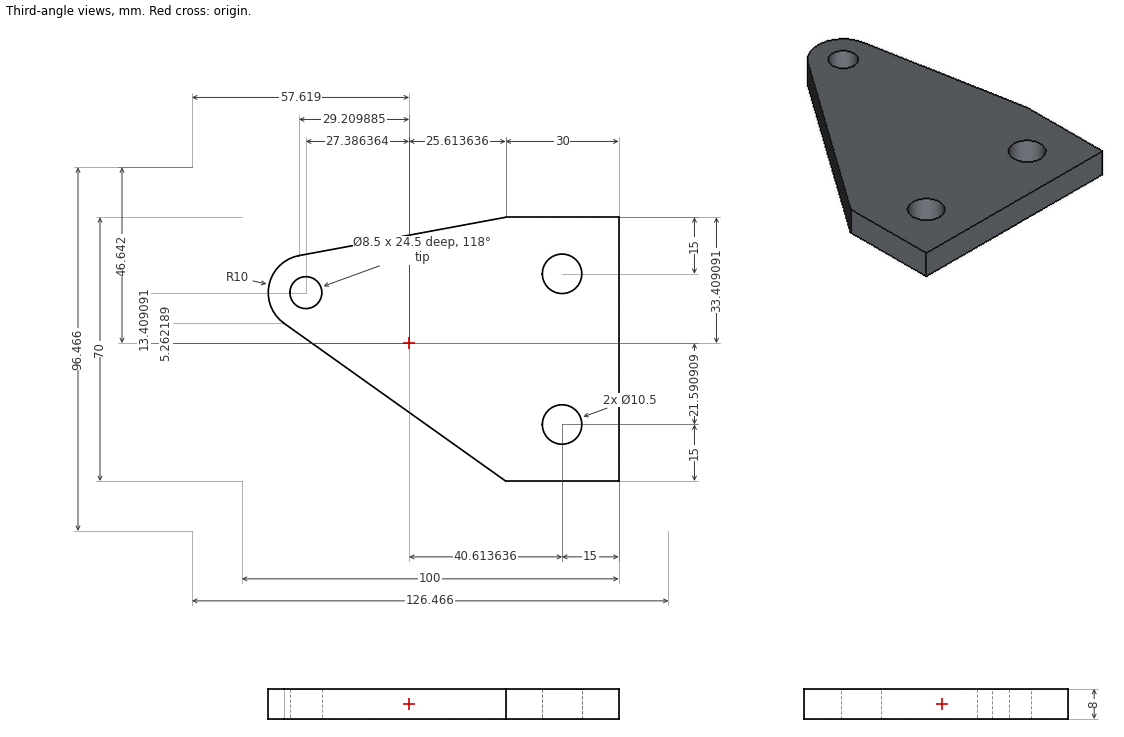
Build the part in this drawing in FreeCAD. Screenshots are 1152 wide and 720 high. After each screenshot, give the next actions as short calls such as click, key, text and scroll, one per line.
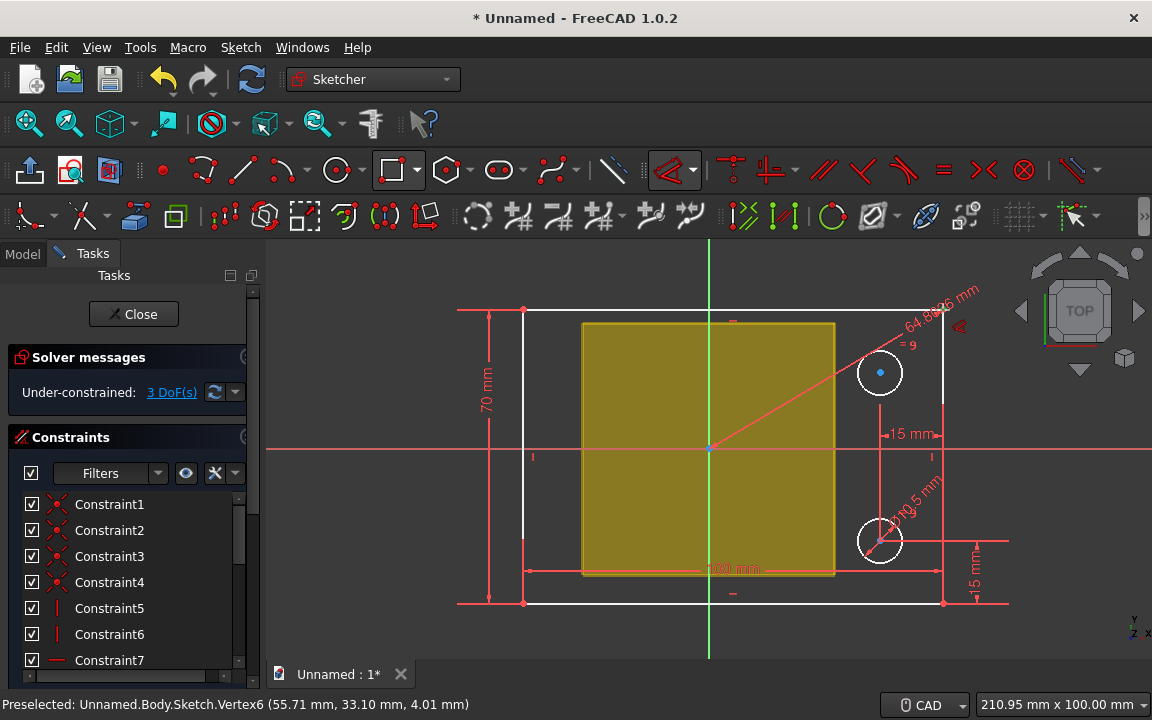
click(880, 373)
click(912, 276)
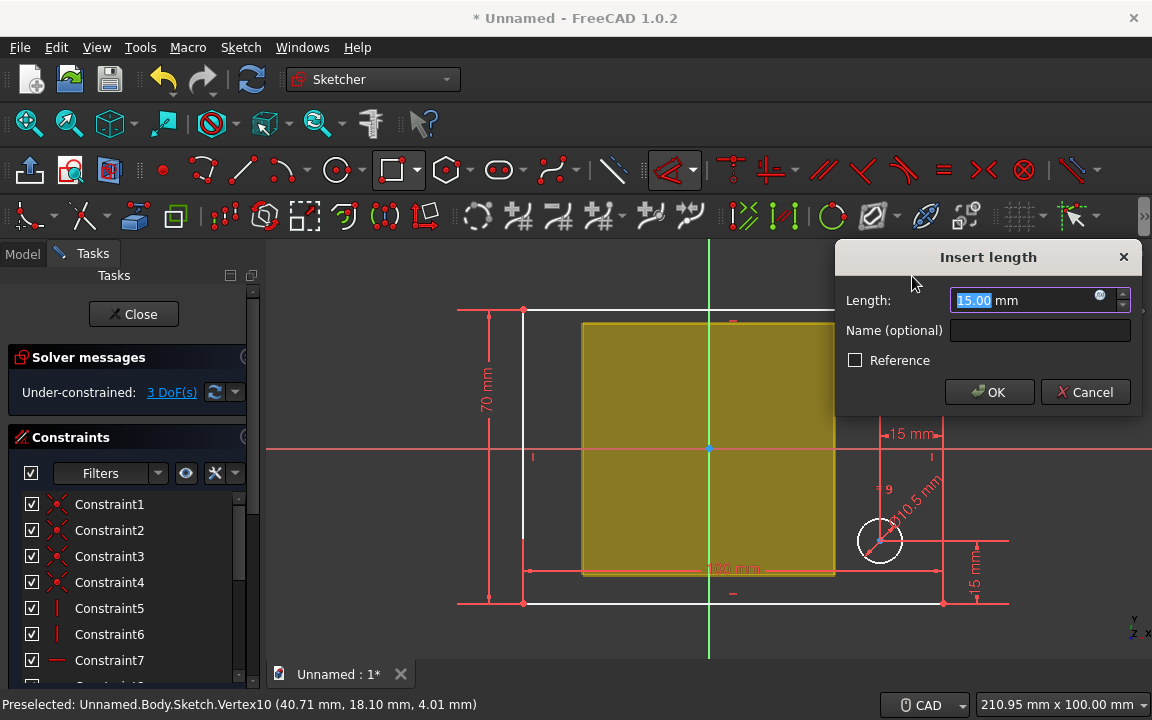
text(15)
key(Return)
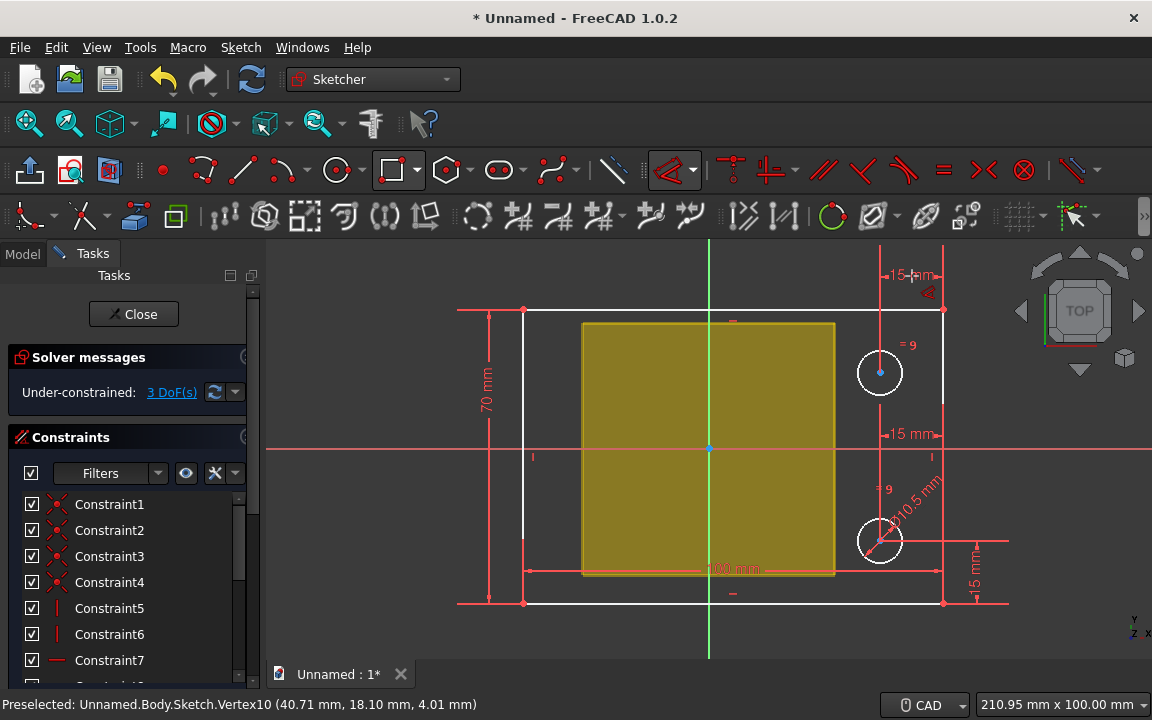
click(943, 310)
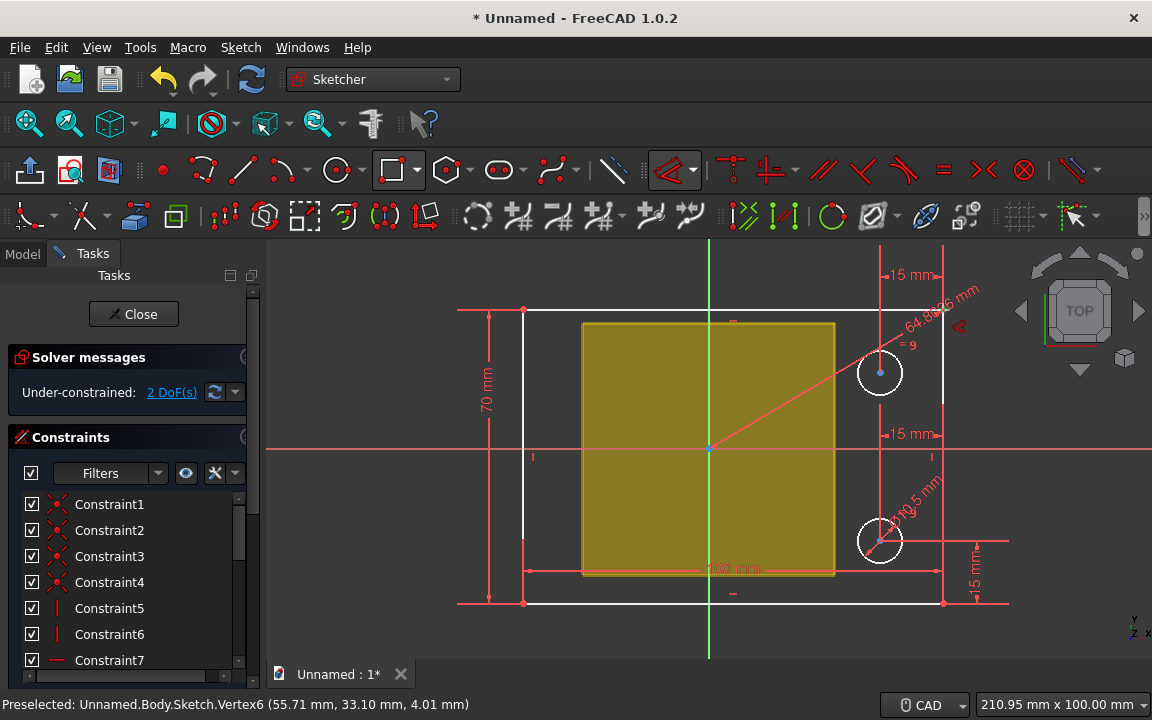
click(880, 373)
click(977, 341)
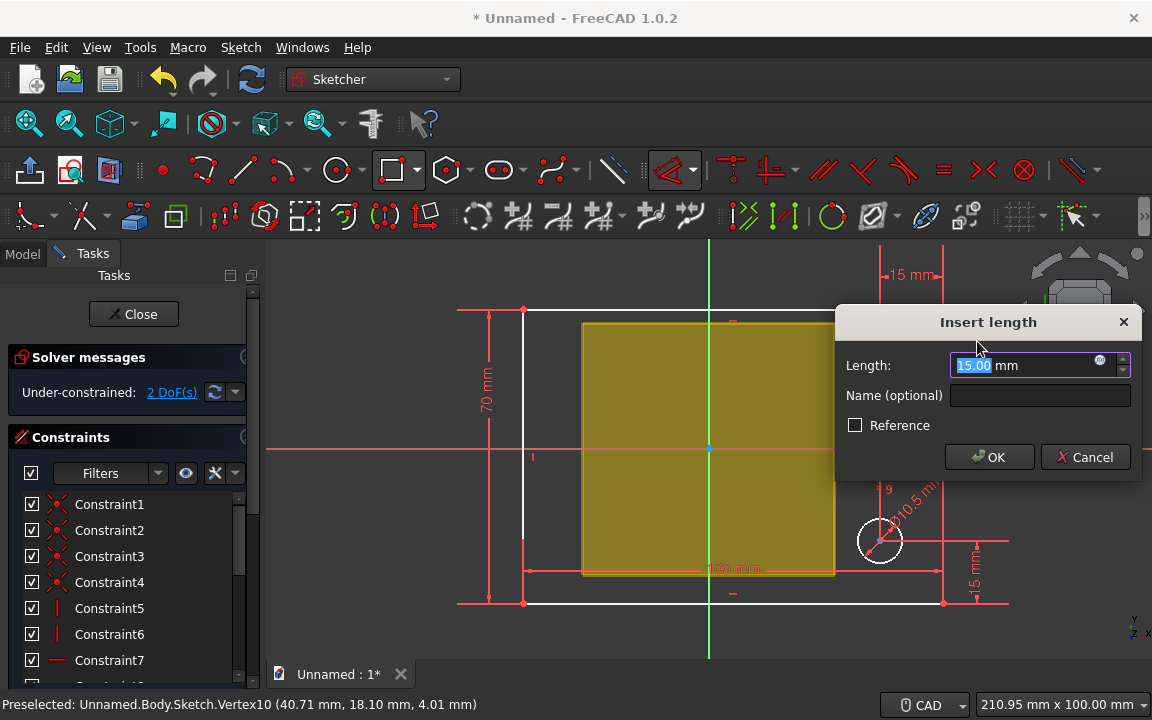
text(15)
key(Return)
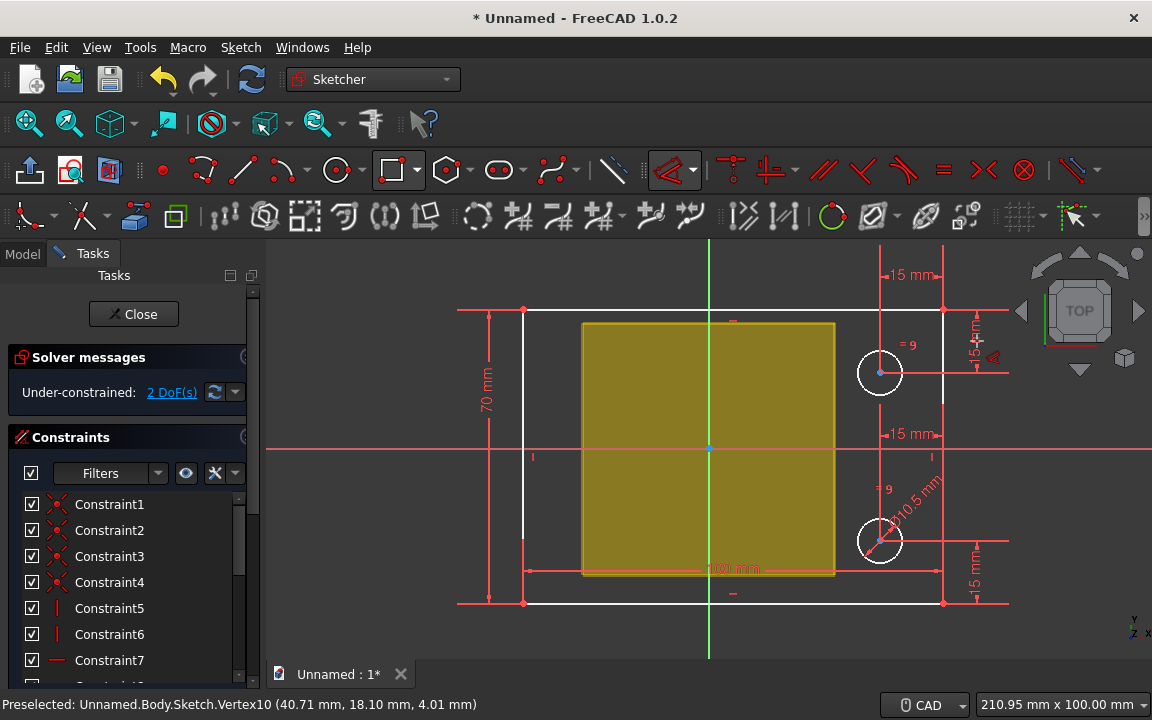
click(880, 541)
click(834, 575)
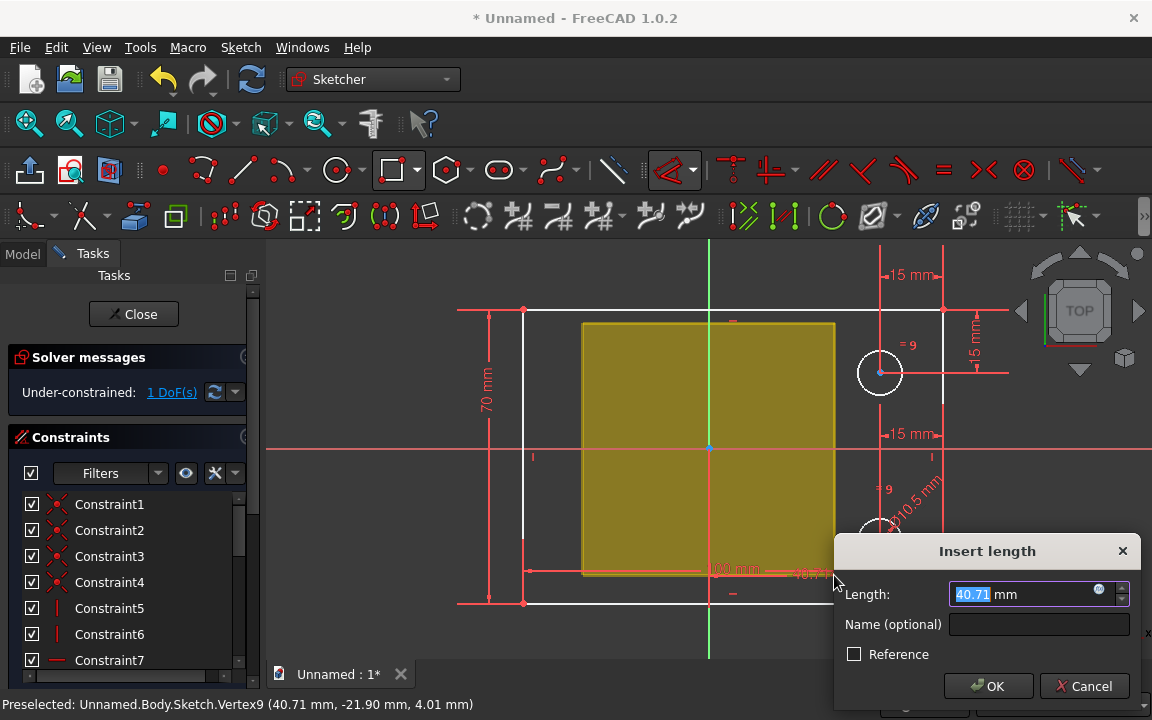
text(40.613636)
key(Return)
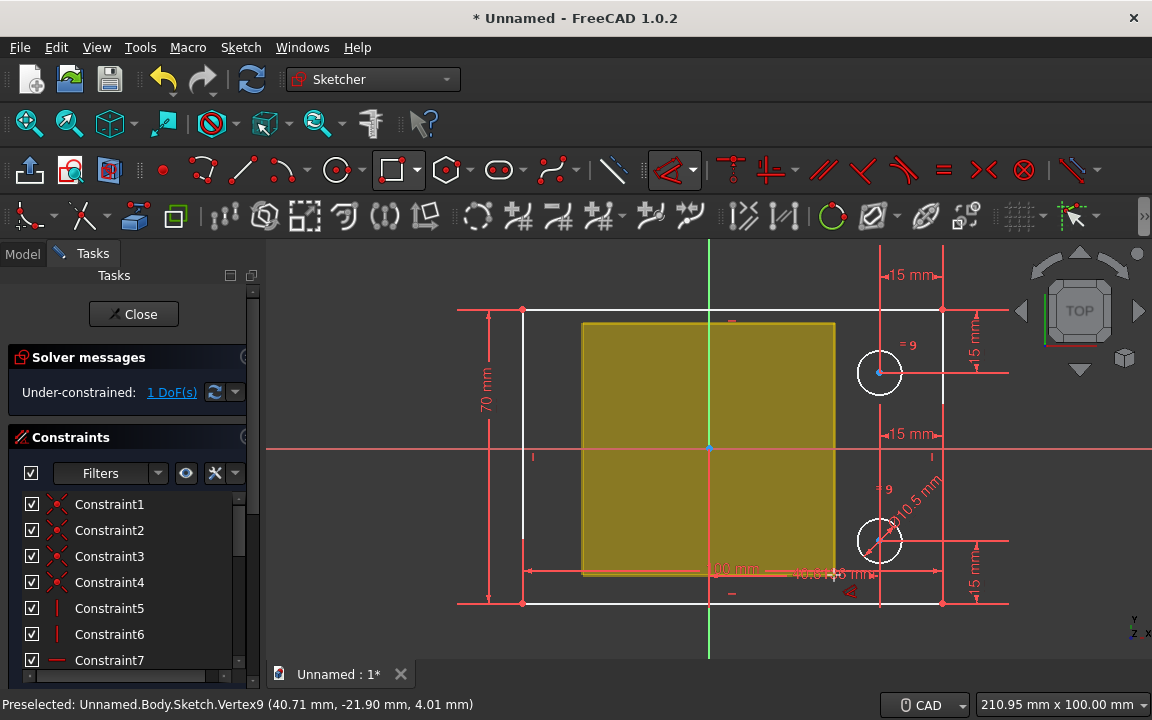
click(880, 541)
click(914, 474)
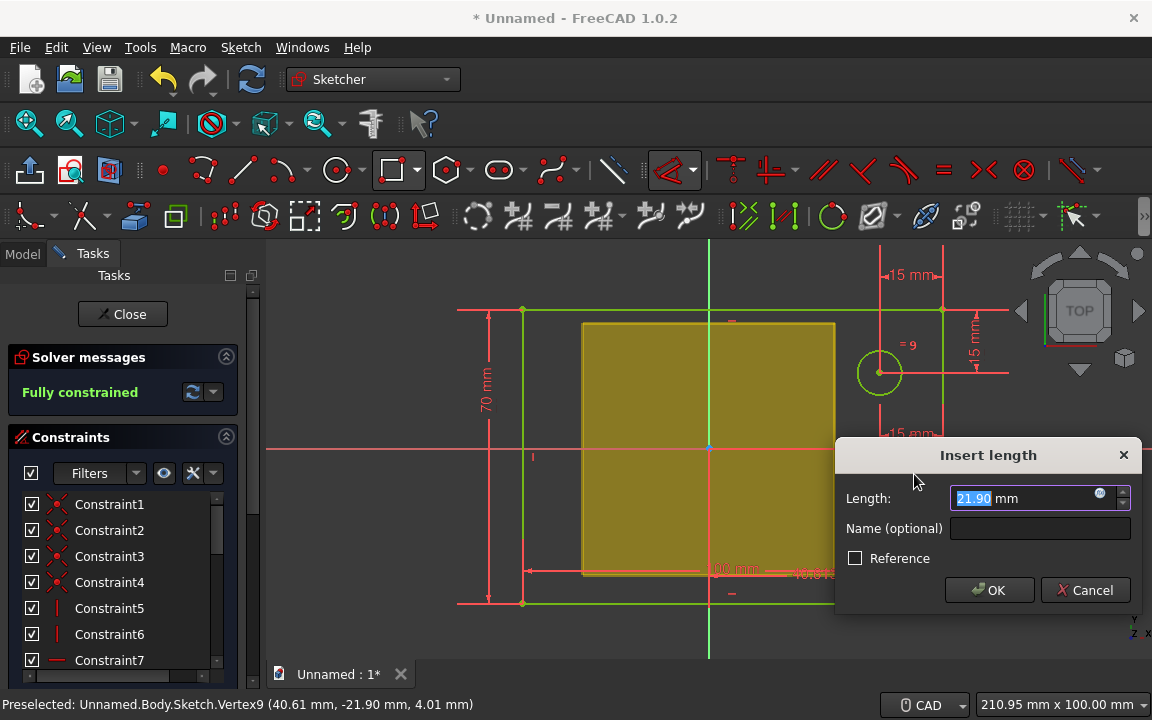
text(21.590909)
key(Return)
key(Escape)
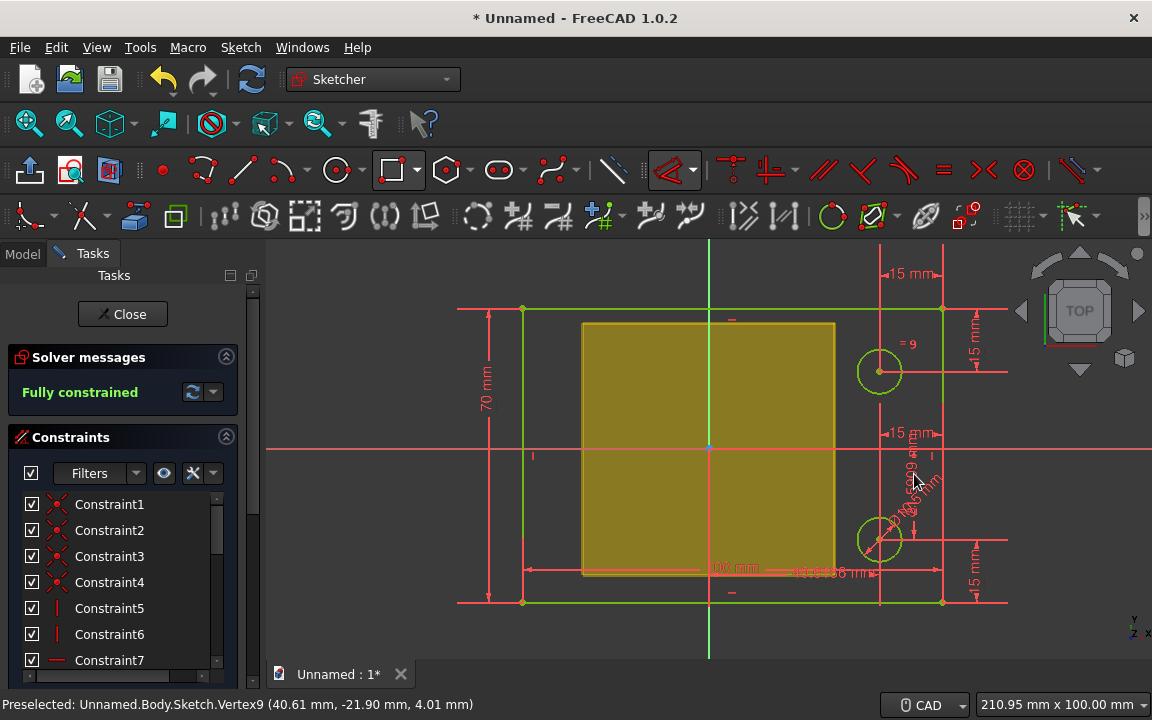
click(123, 314)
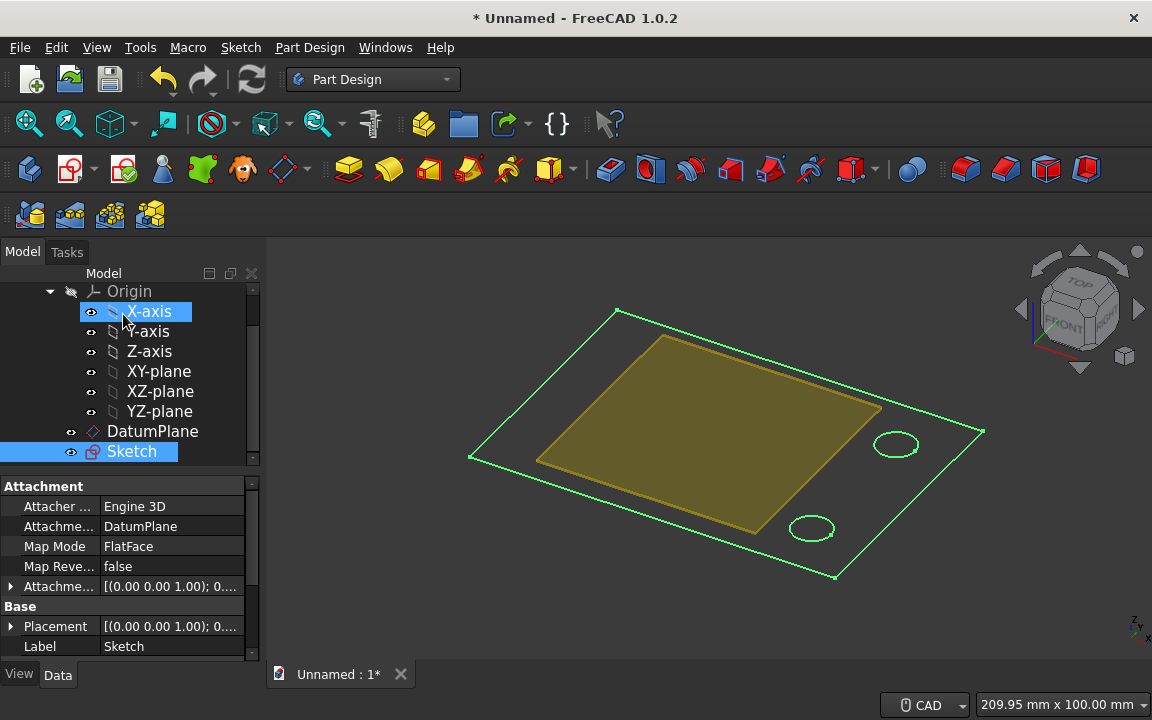
click(350, 170)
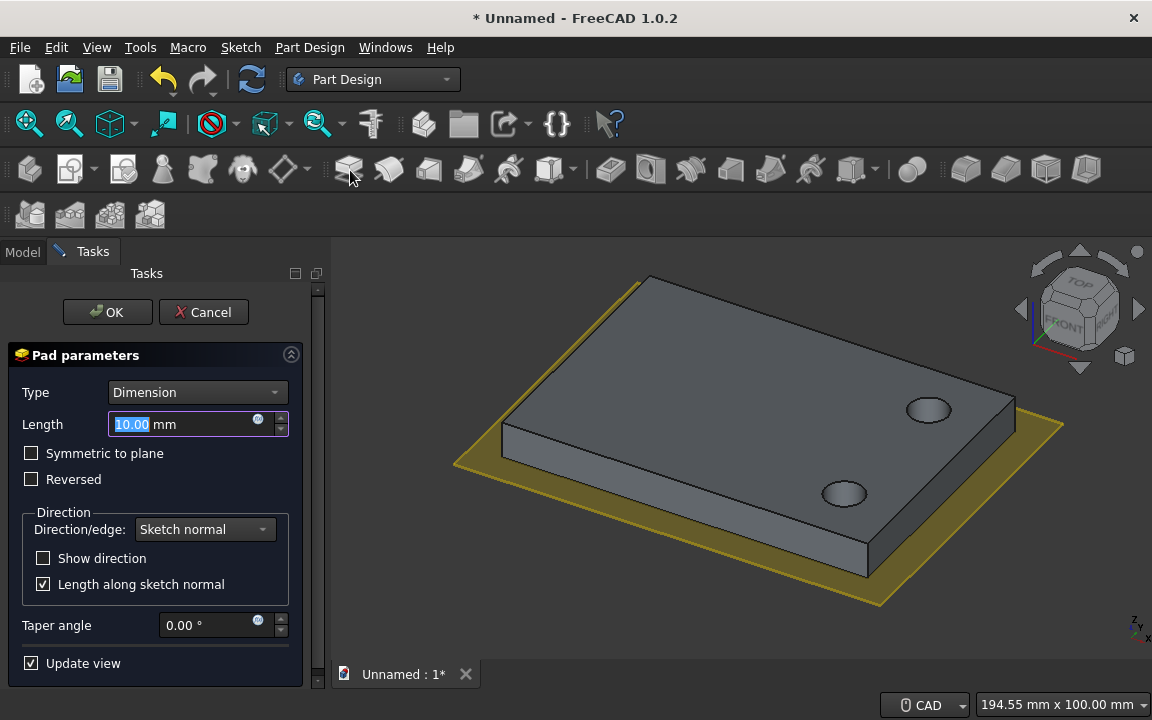
text(8)
key(Tab)